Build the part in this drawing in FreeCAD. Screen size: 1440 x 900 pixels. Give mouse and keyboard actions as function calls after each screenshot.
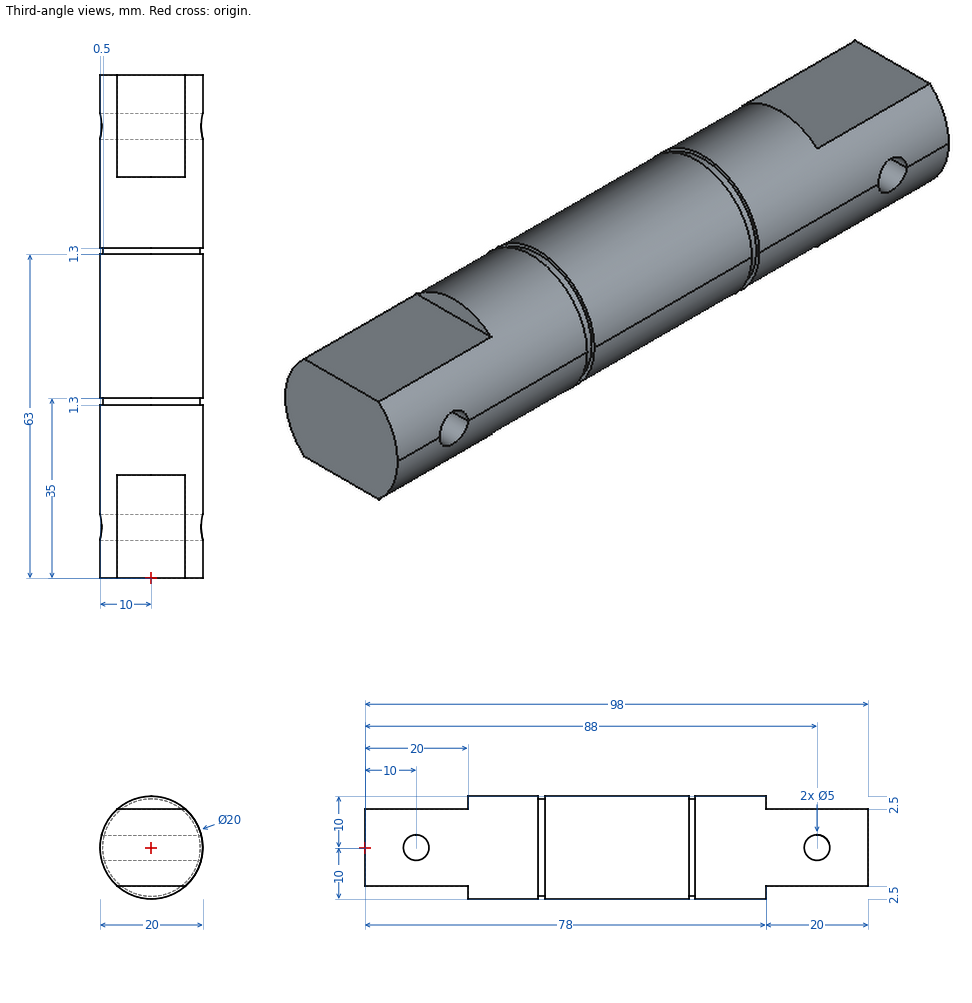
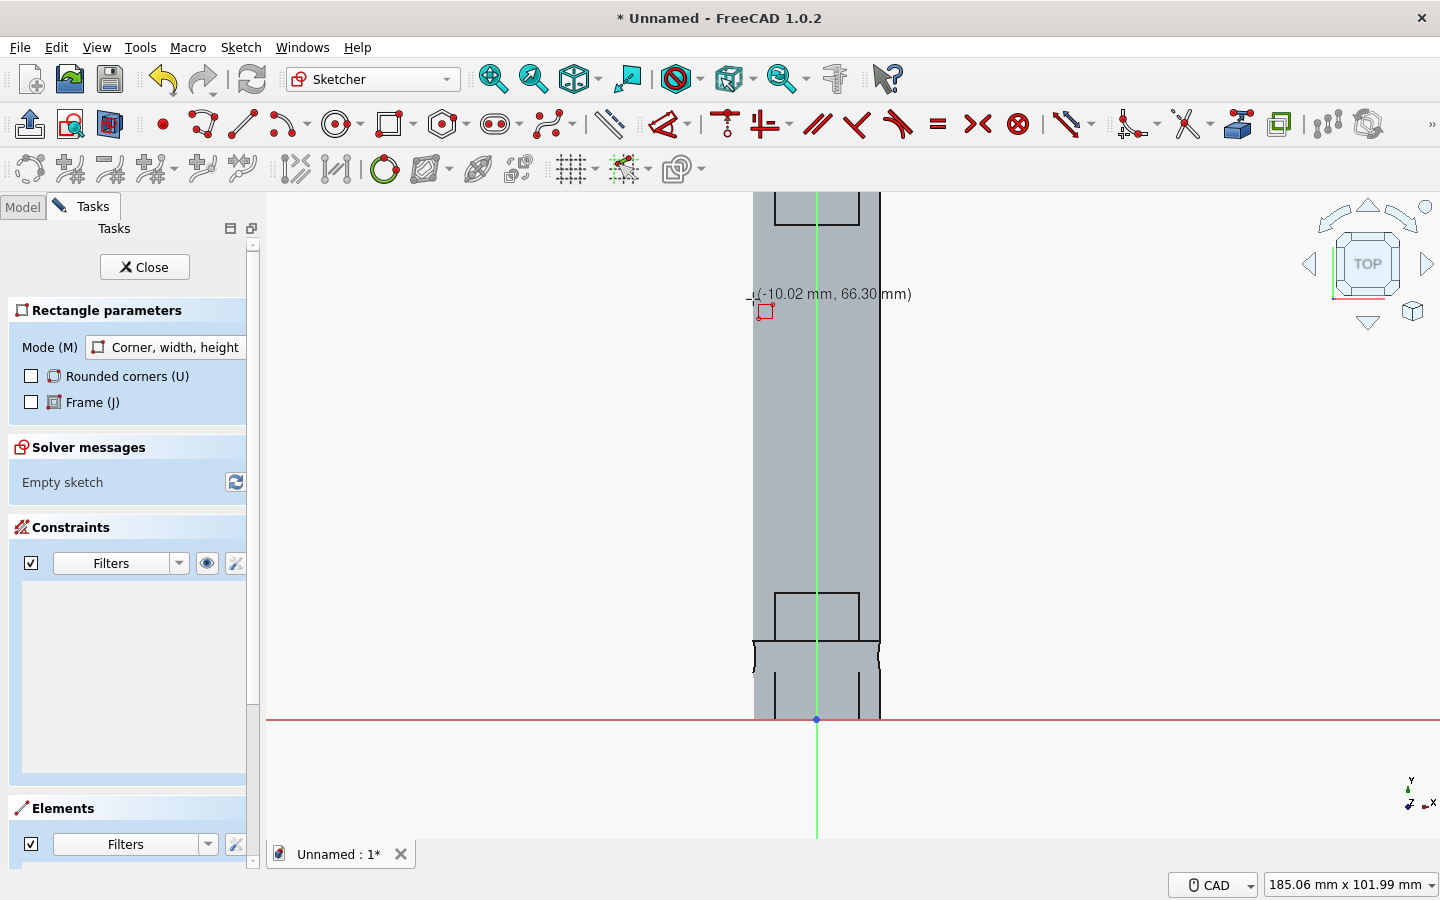
click(753, 312)
move(757, 320)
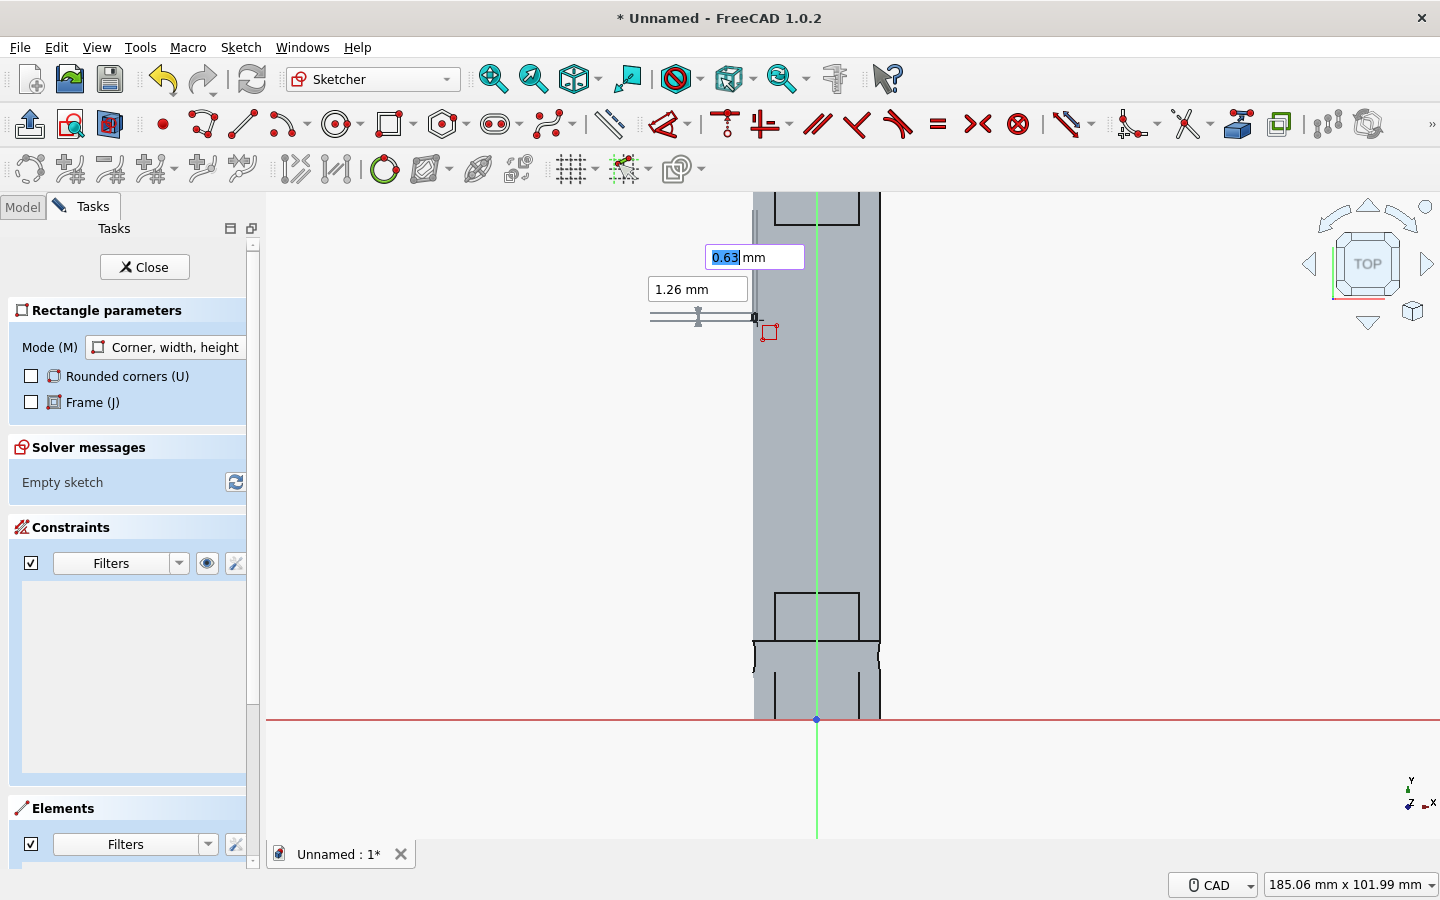
text(0.5)
key(Tab)
text(1.3)
key(Return)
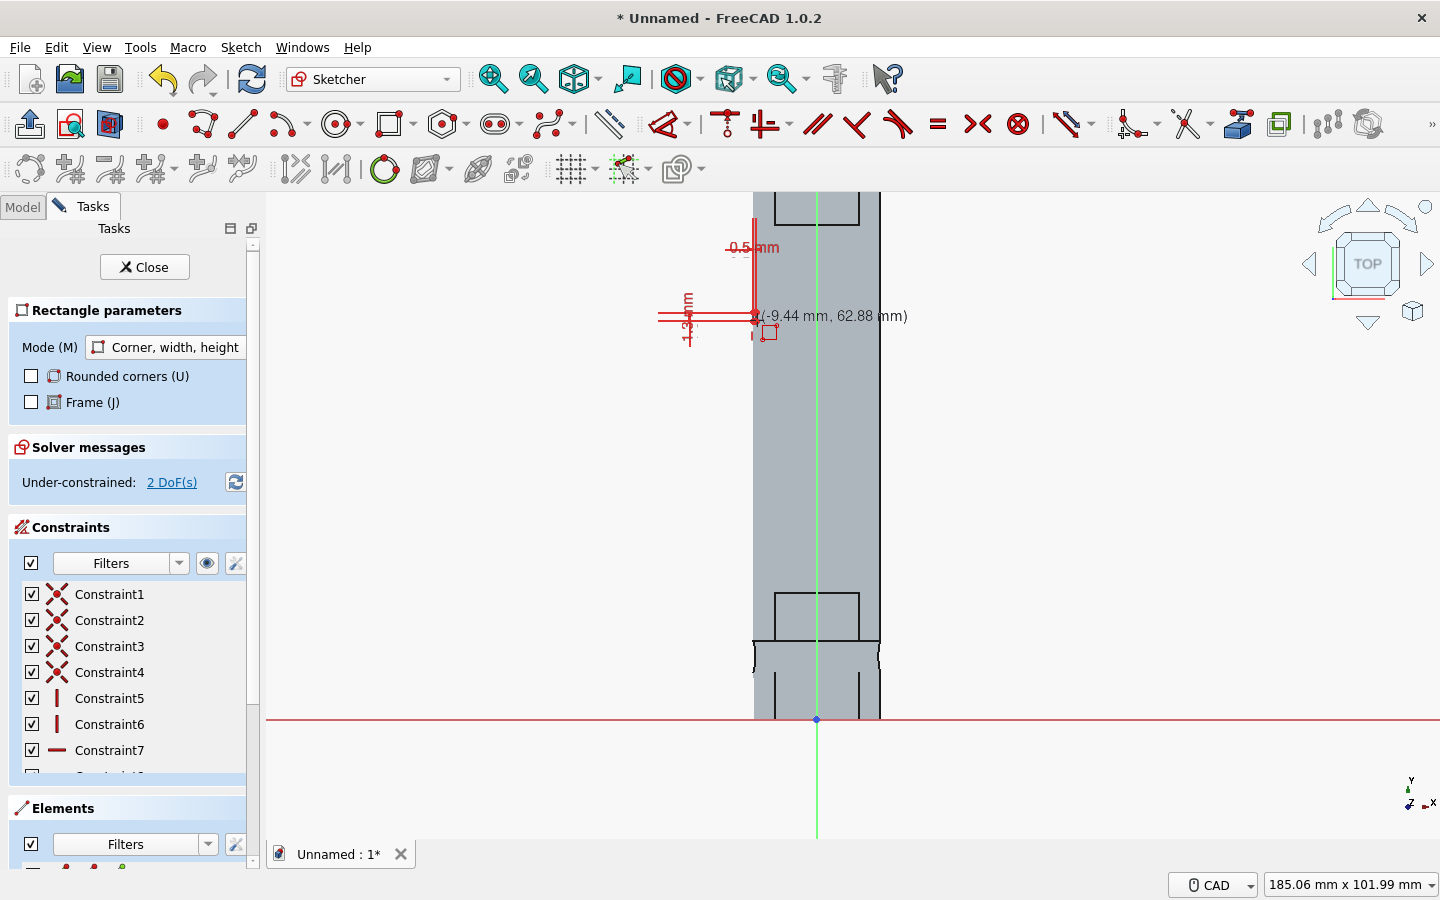
scroll(753, 498, up, 9)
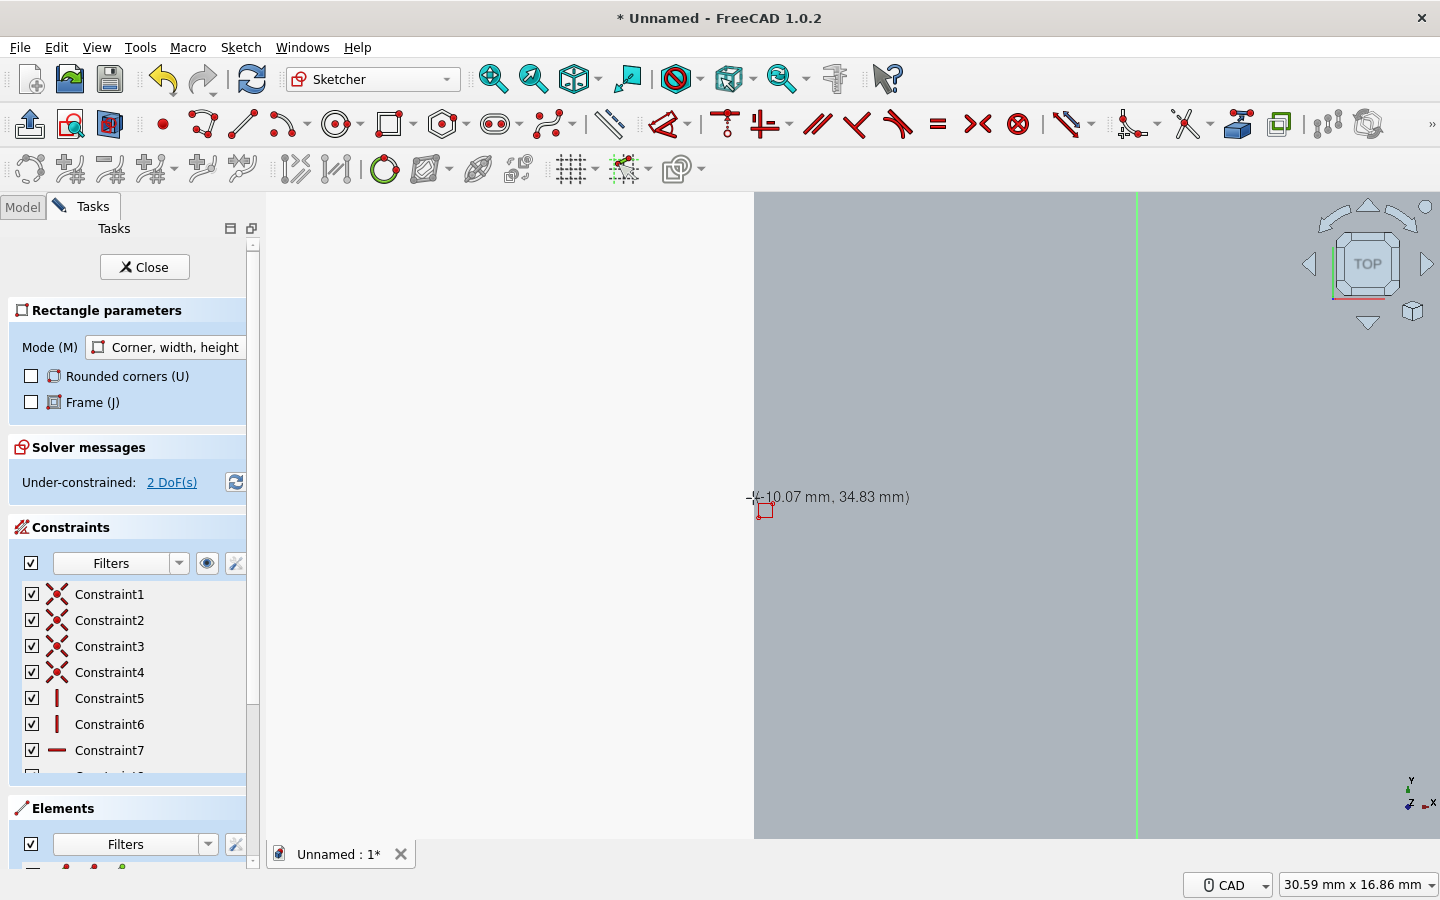
scroll(753, 498, down, 9)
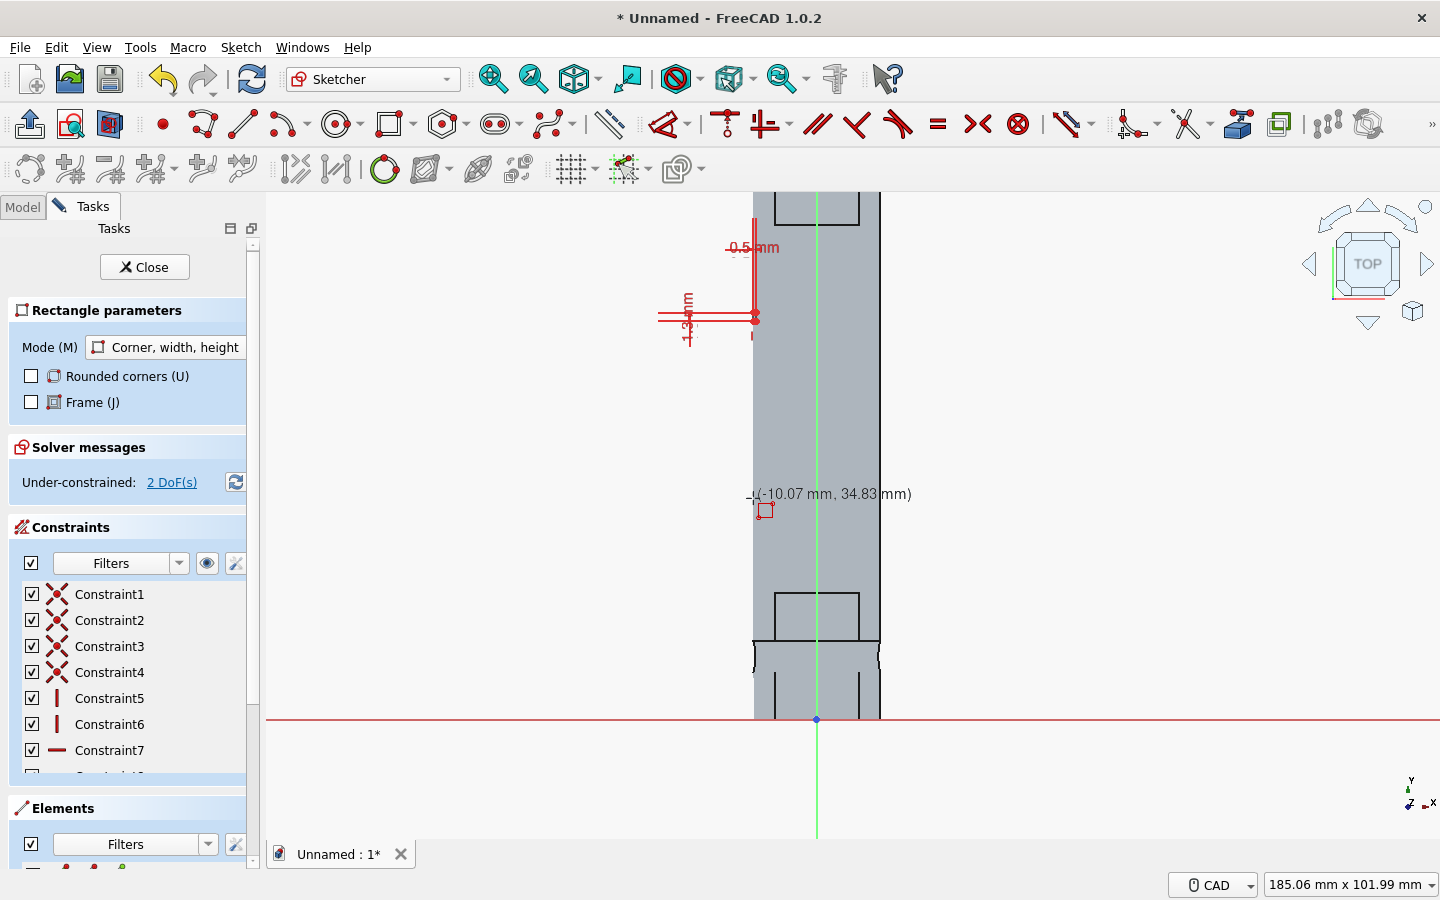
click(753, 498)
move(757, 506)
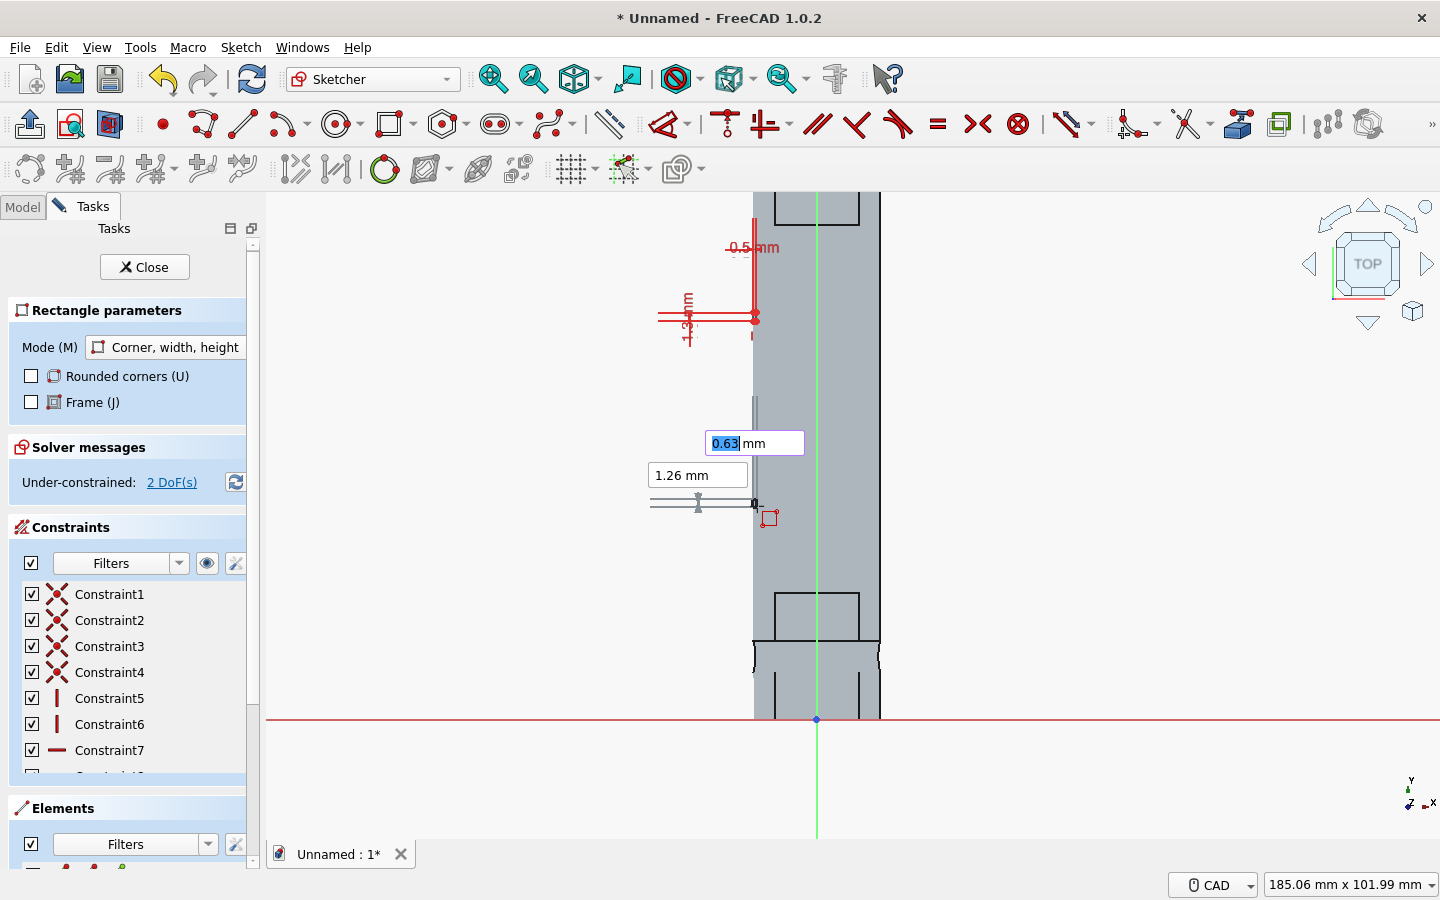
text(0.5)
key(Tab)
text(1.3)
key(Return)
key(Escape)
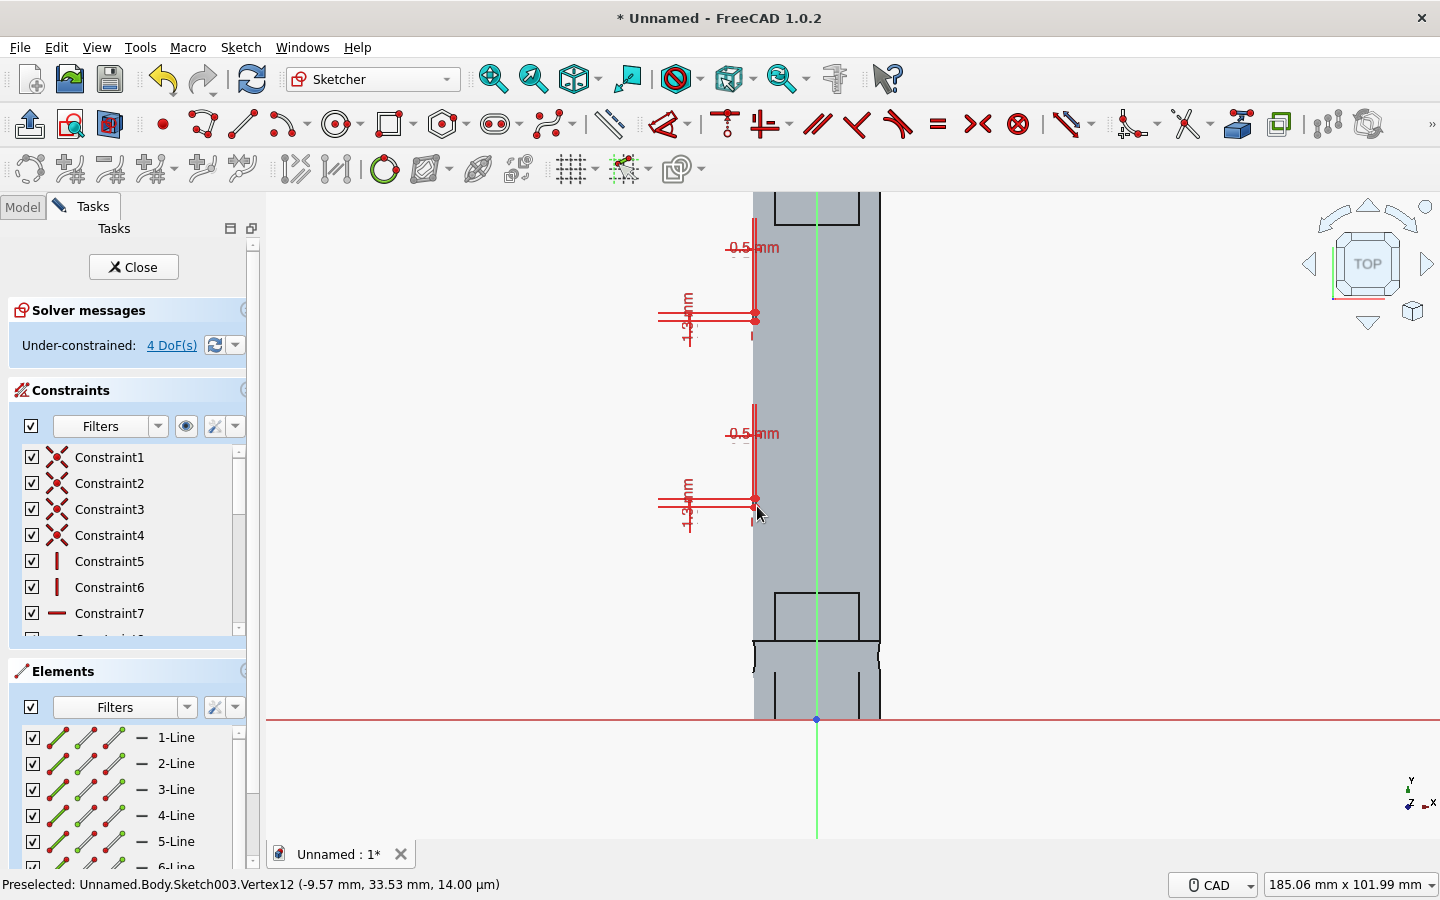
click(664, 124)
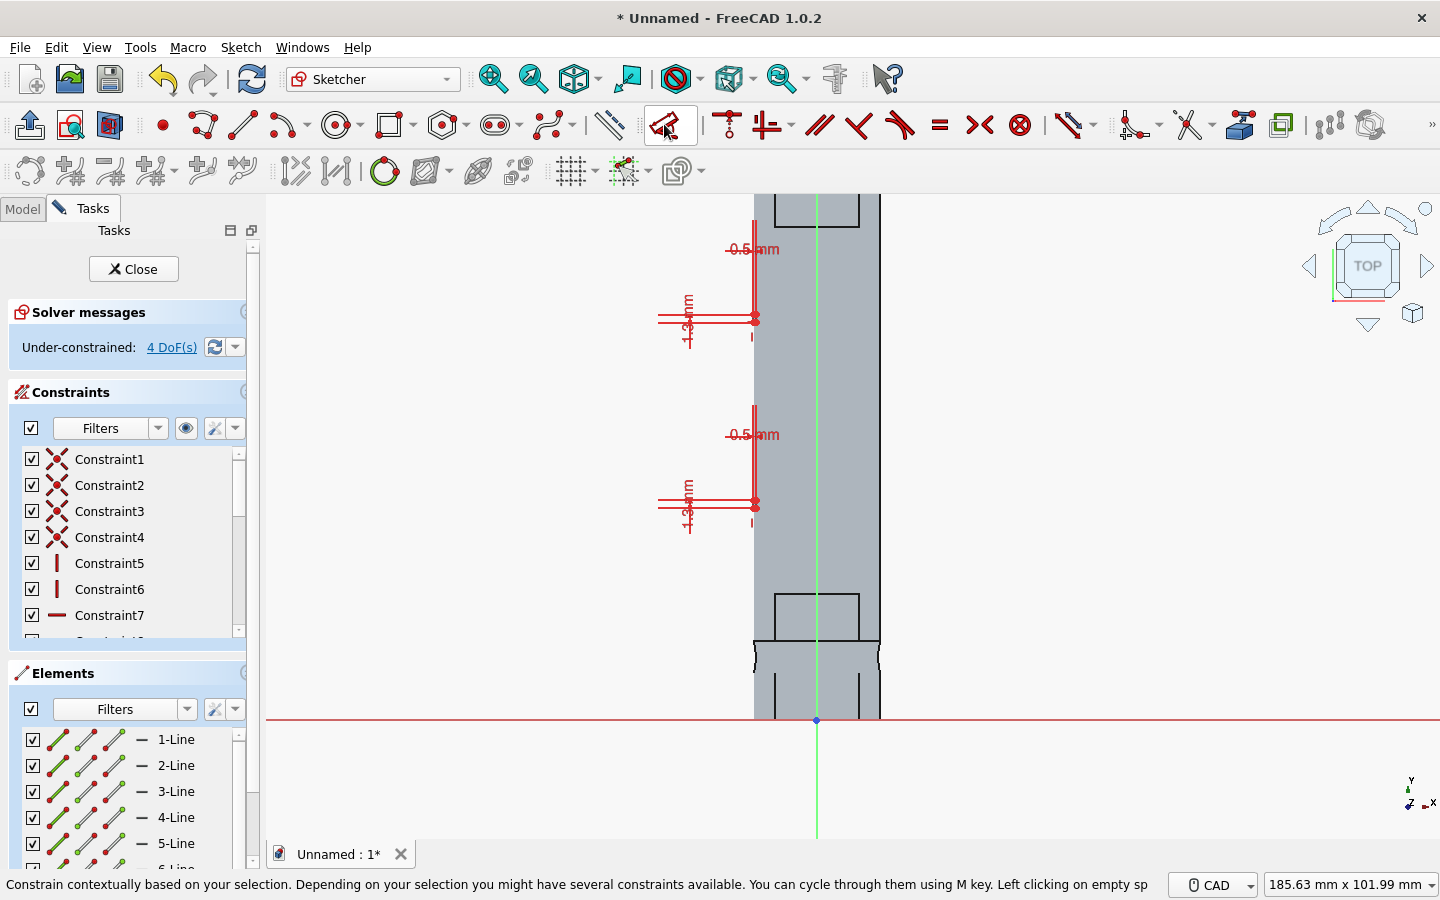
scroll(753, 315, up, 7)